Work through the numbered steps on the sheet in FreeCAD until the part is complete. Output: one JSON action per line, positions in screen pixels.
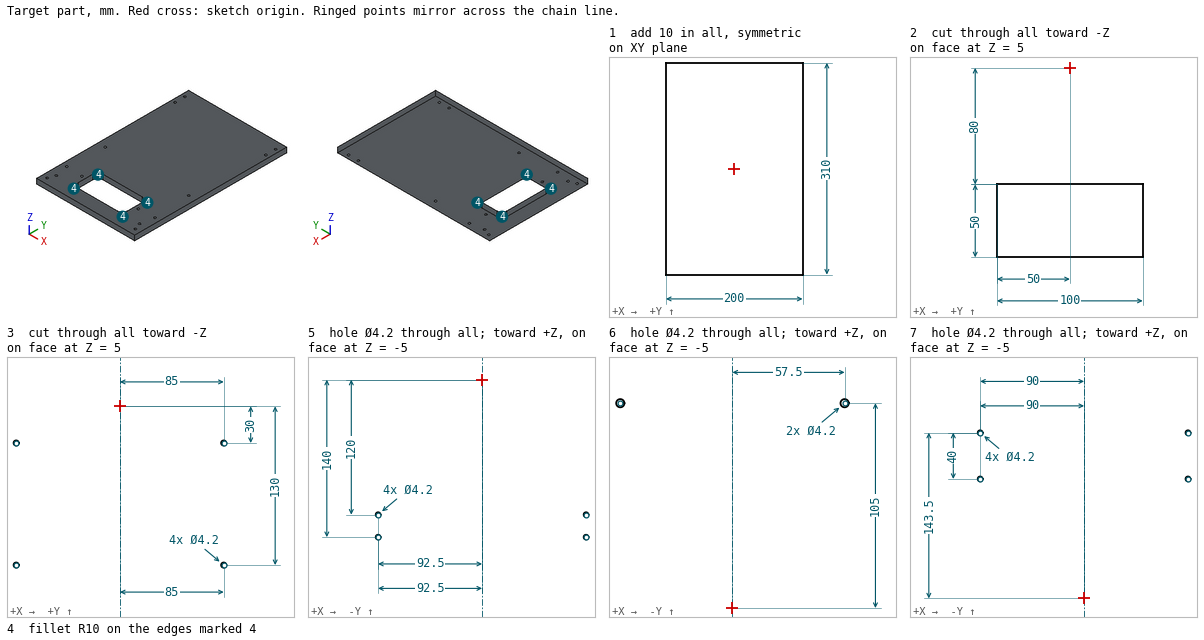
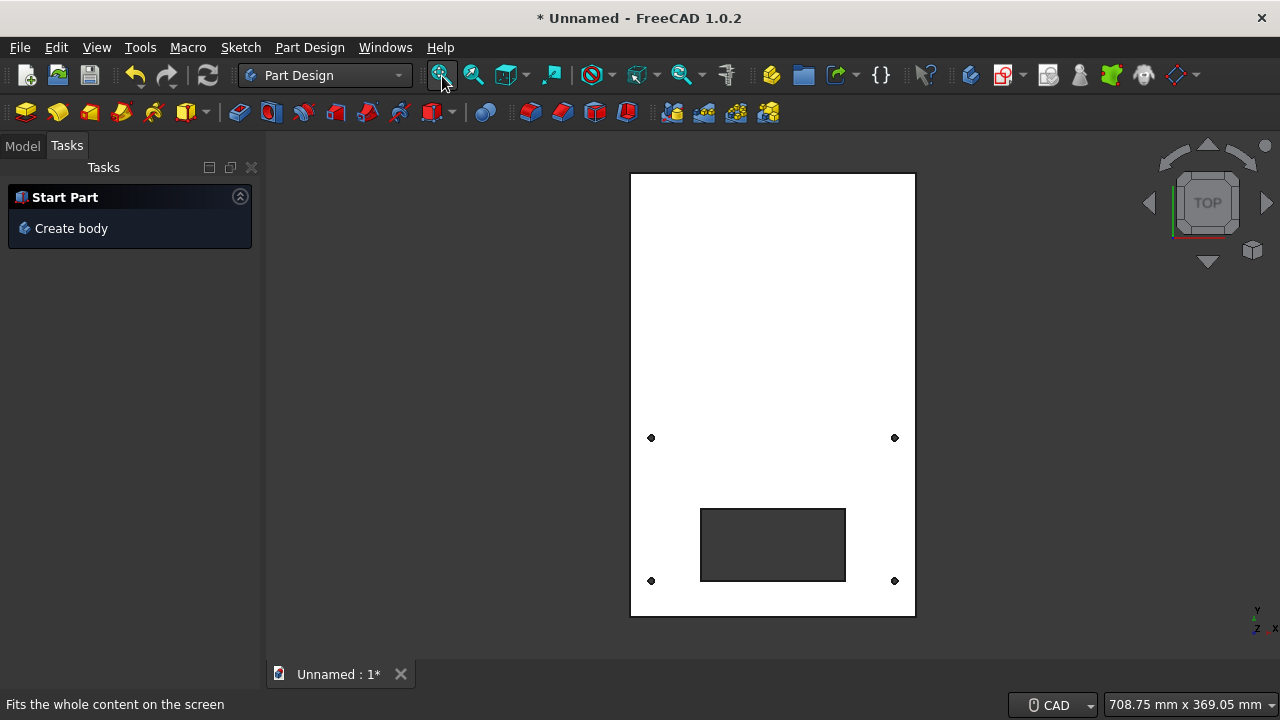
{"action": "scroll", "coordinate": [845, 508], "scroll_direction": "up", "scroll_amount": 6}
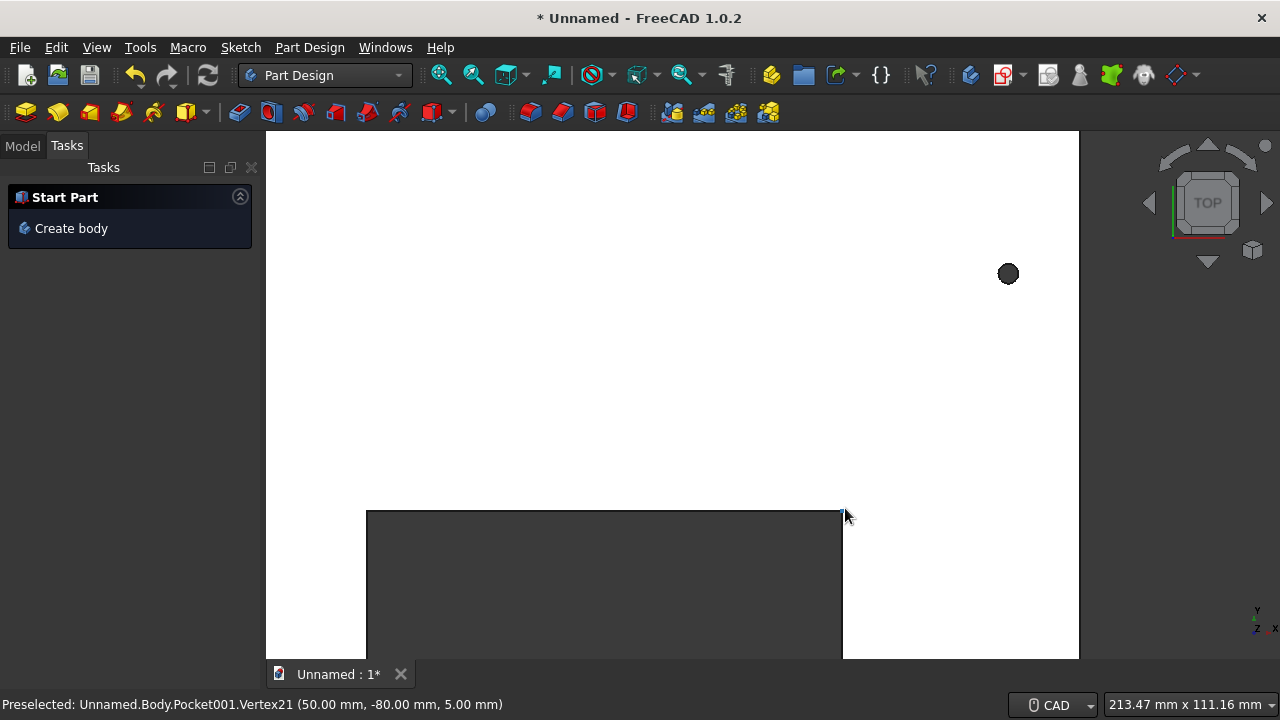
{"action": "left_click", "coordinate": [442, 76]}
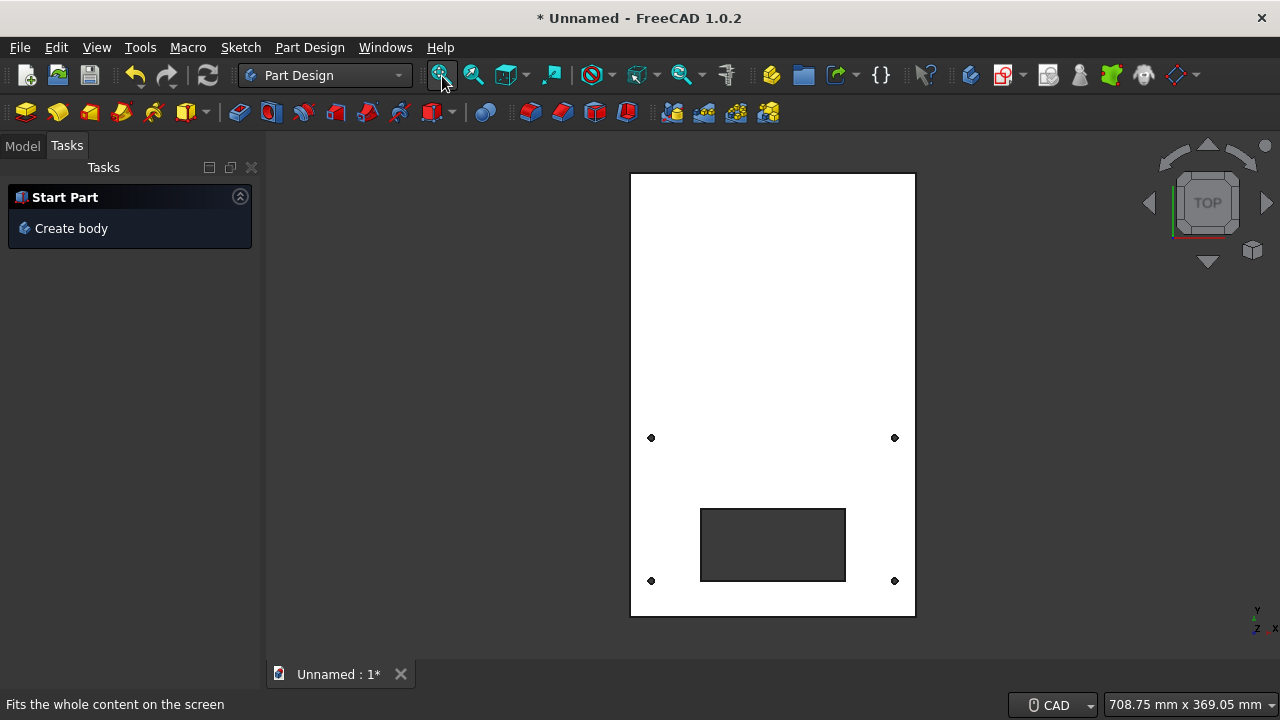
{"action": "key", "text": "1"}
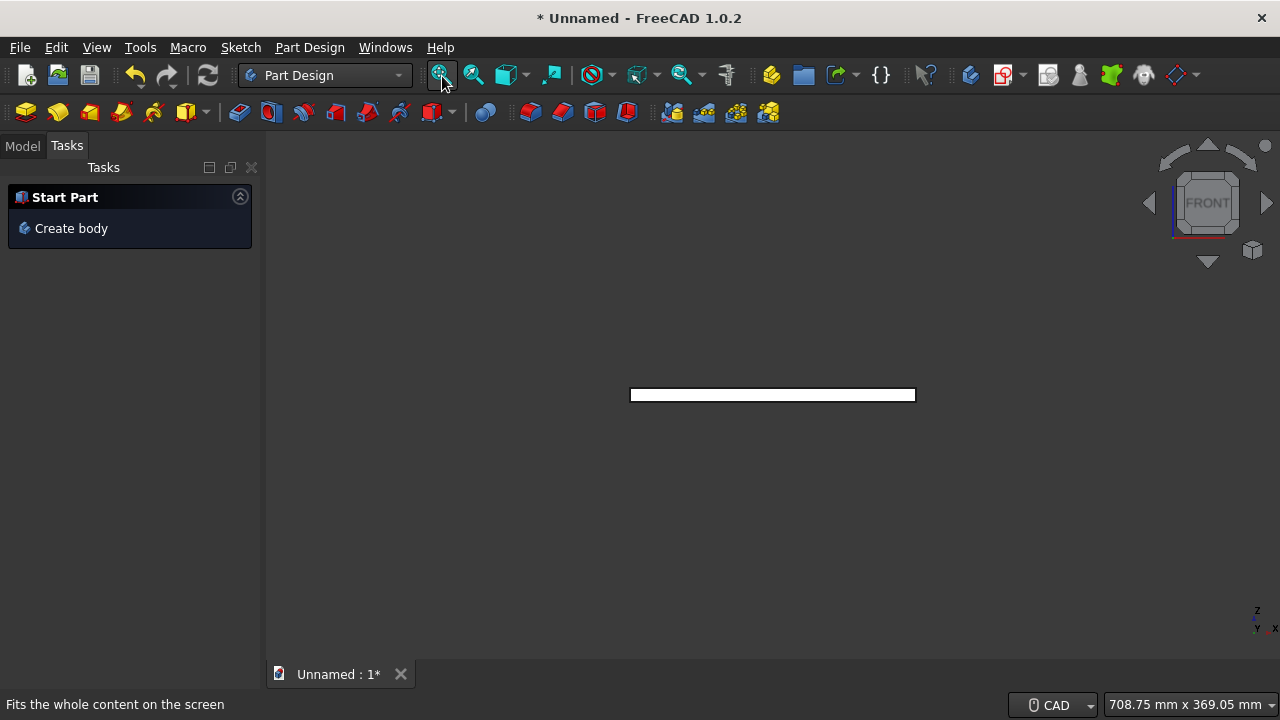
{"action": "left_click", "coordinate": [442, 76]}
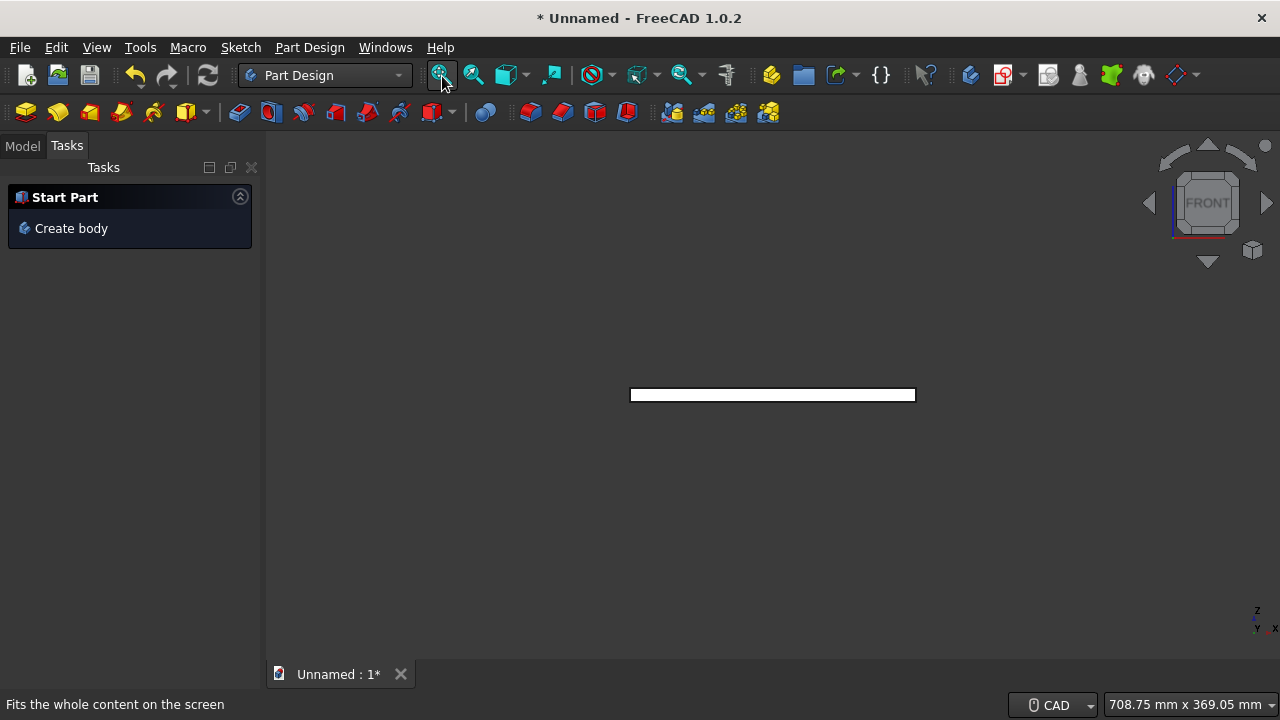
{"action": "scroll", "coordinate": [845, 394], "scroll_direction": "up", "scroll_amount": 6}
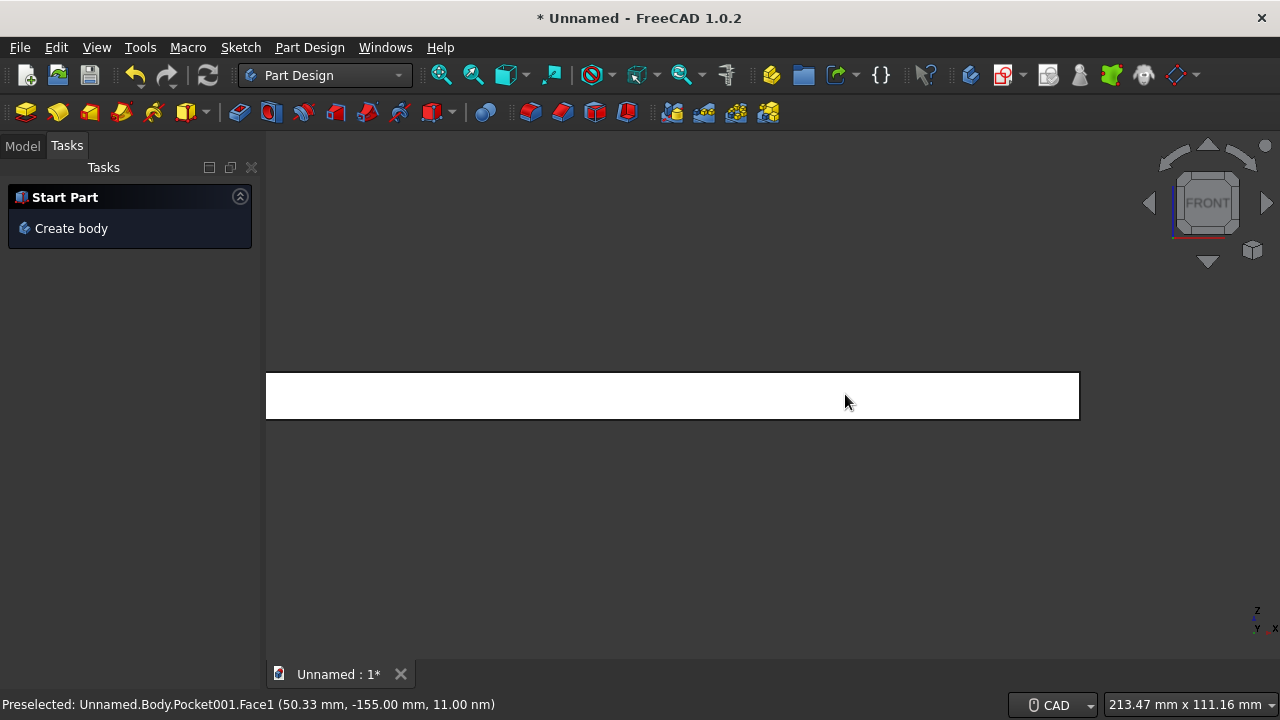
{"action": "left_click", "coordinate": [442, 76]}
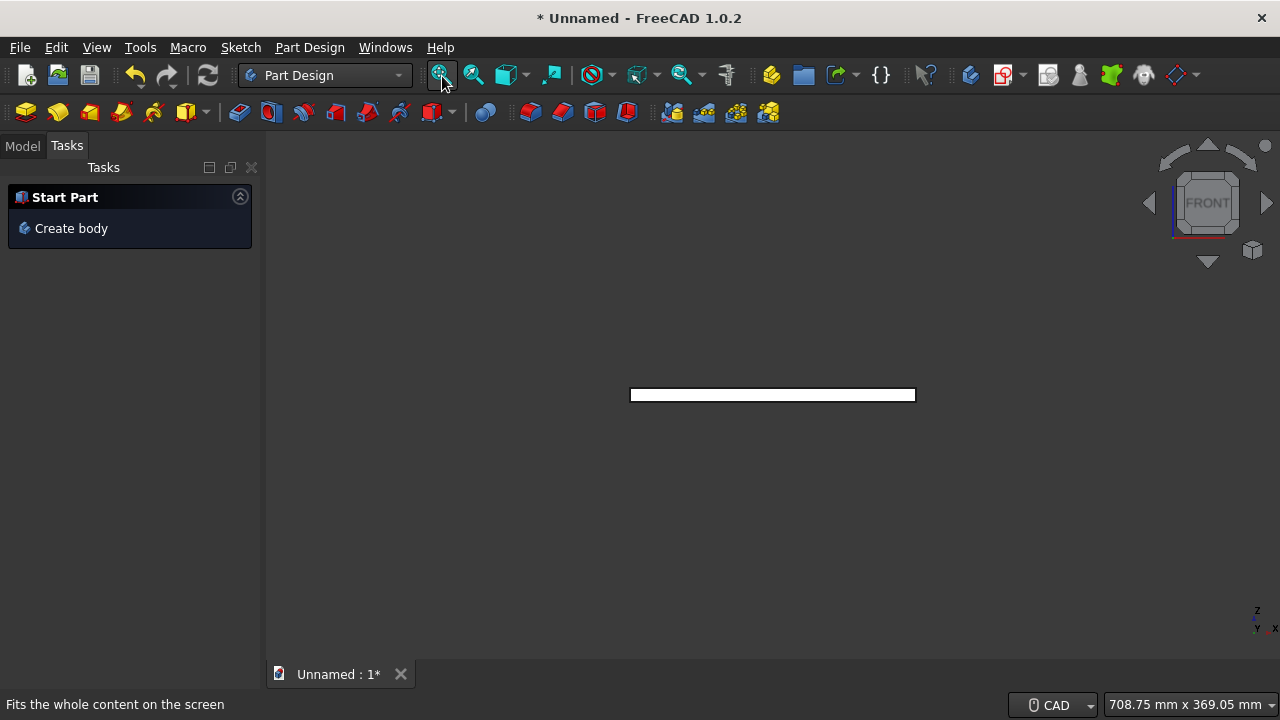
{"action": "key", "text": "3"}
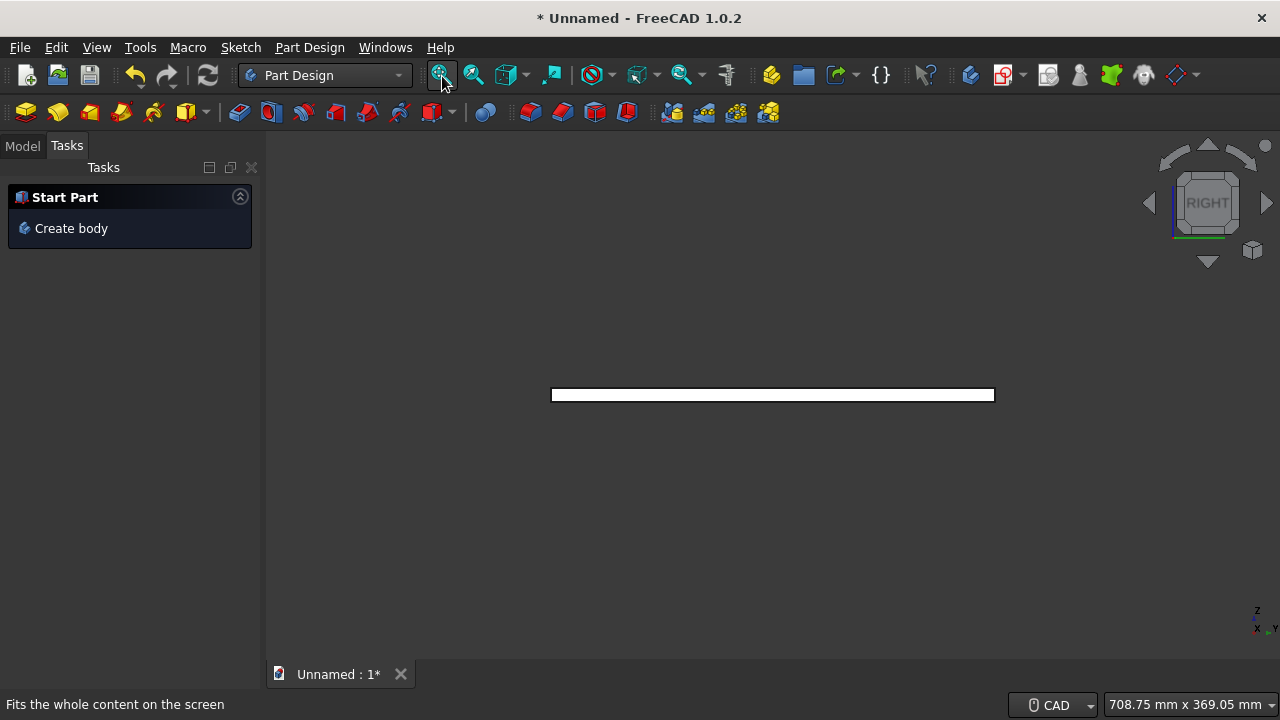
{"action": "left_click", "coordinate": [442, 76]}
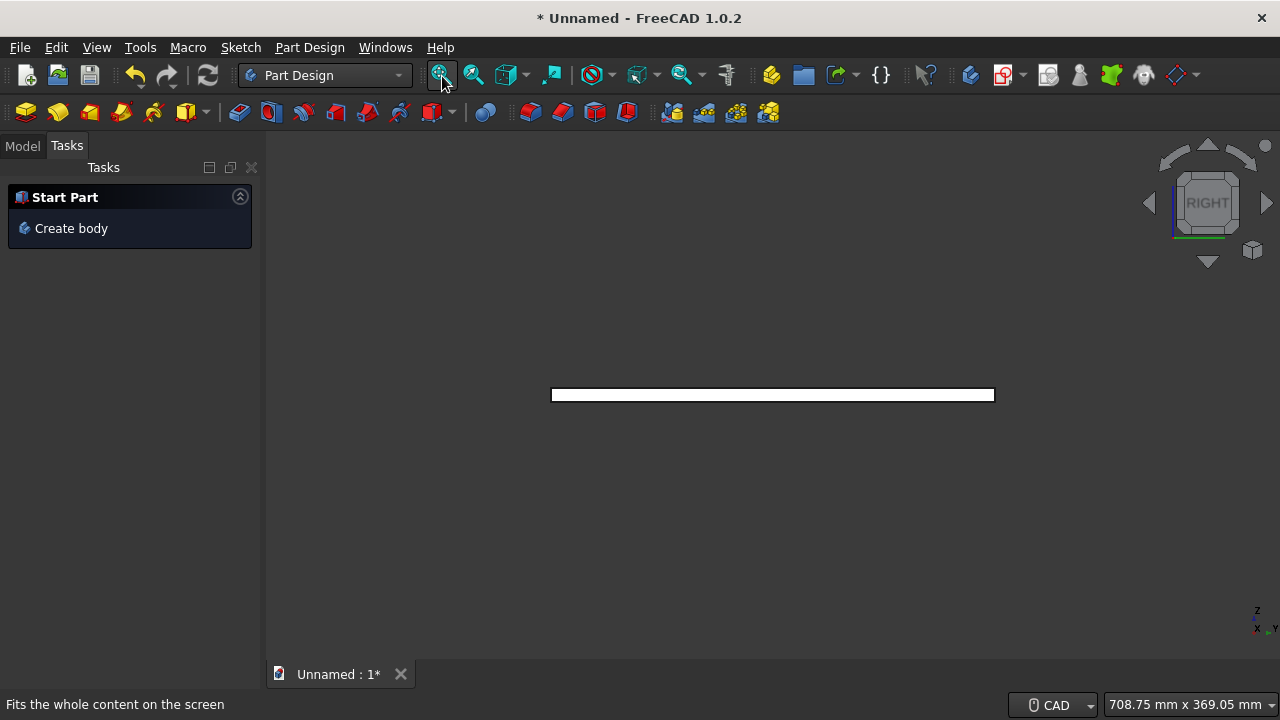
{"action": "scroll", "coordinate": [659, 394], "scroll_direction": "up", "scroll_amount": 6}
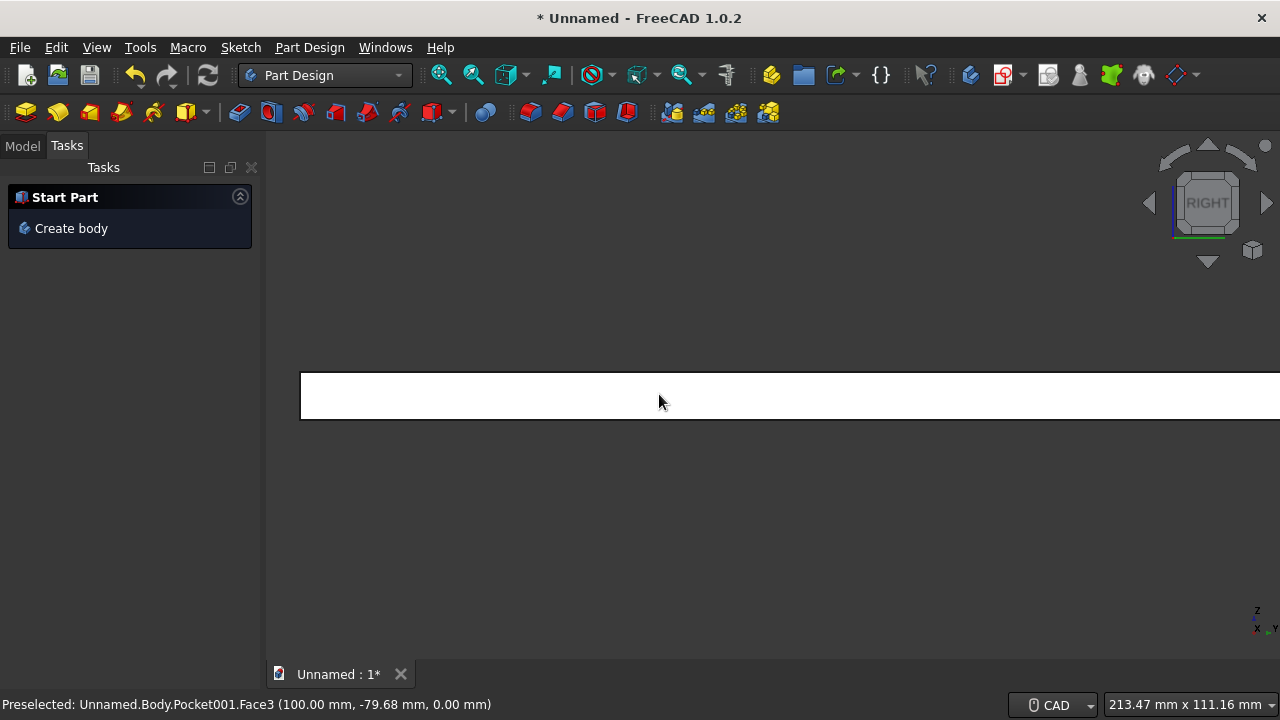
{"action": "left_click", "coordinate": [442, 76]}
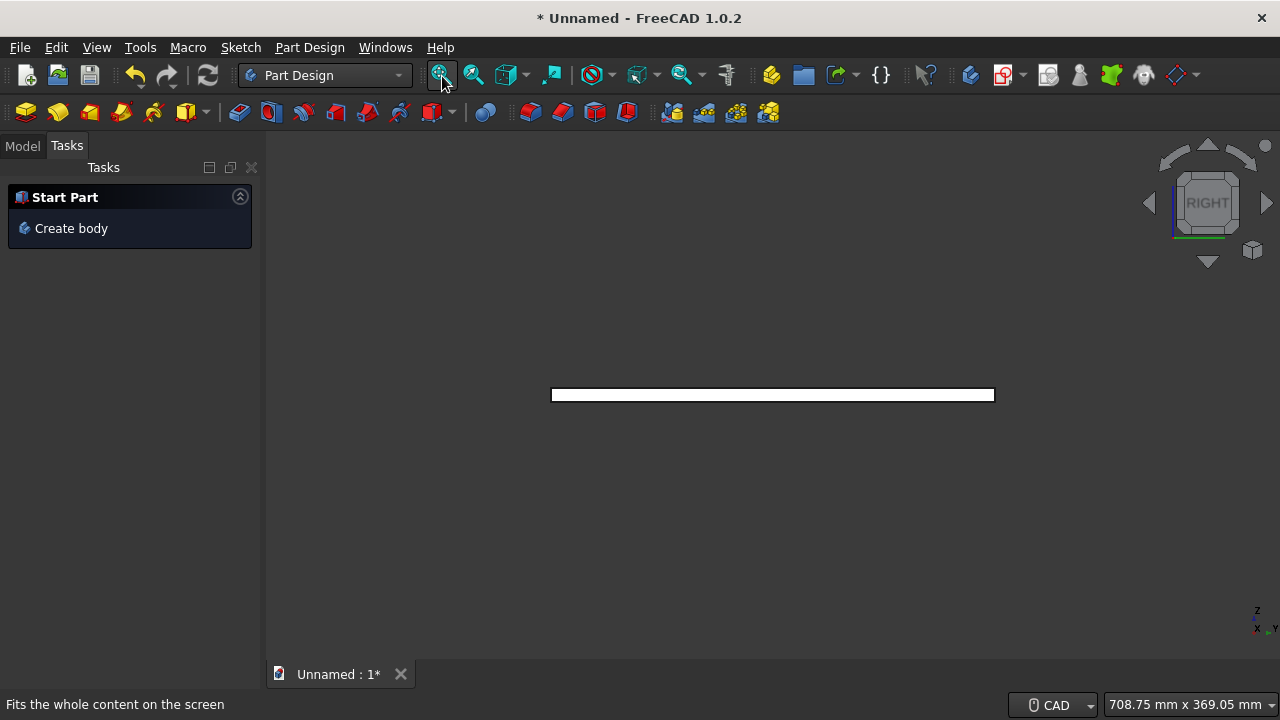
{"action": "key", "text": "5"}